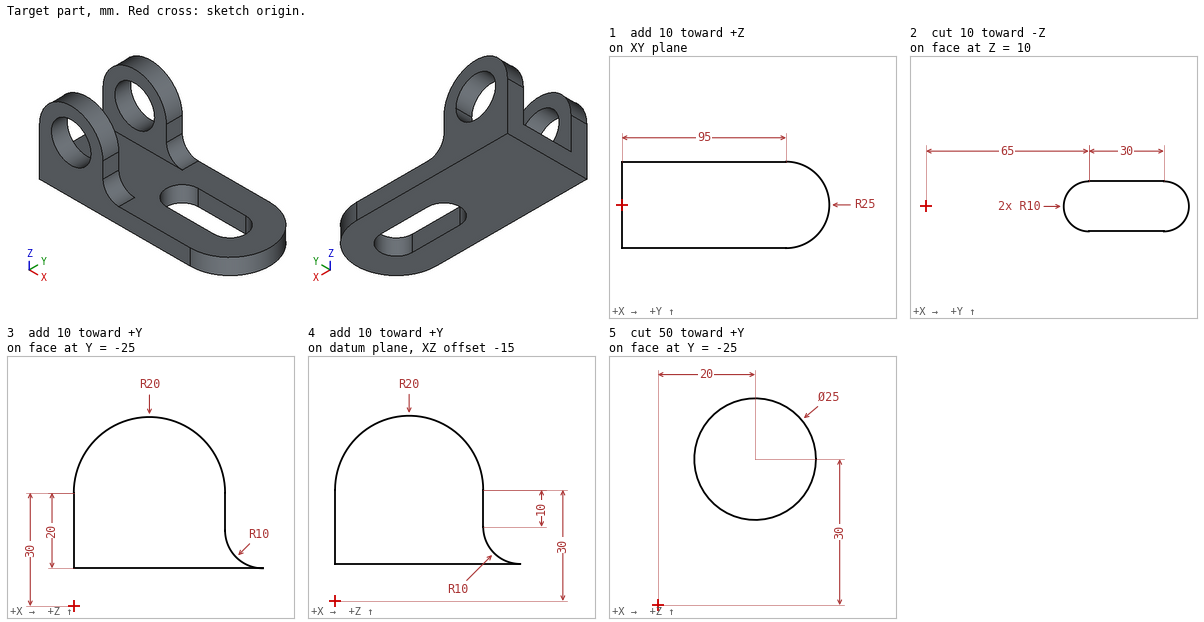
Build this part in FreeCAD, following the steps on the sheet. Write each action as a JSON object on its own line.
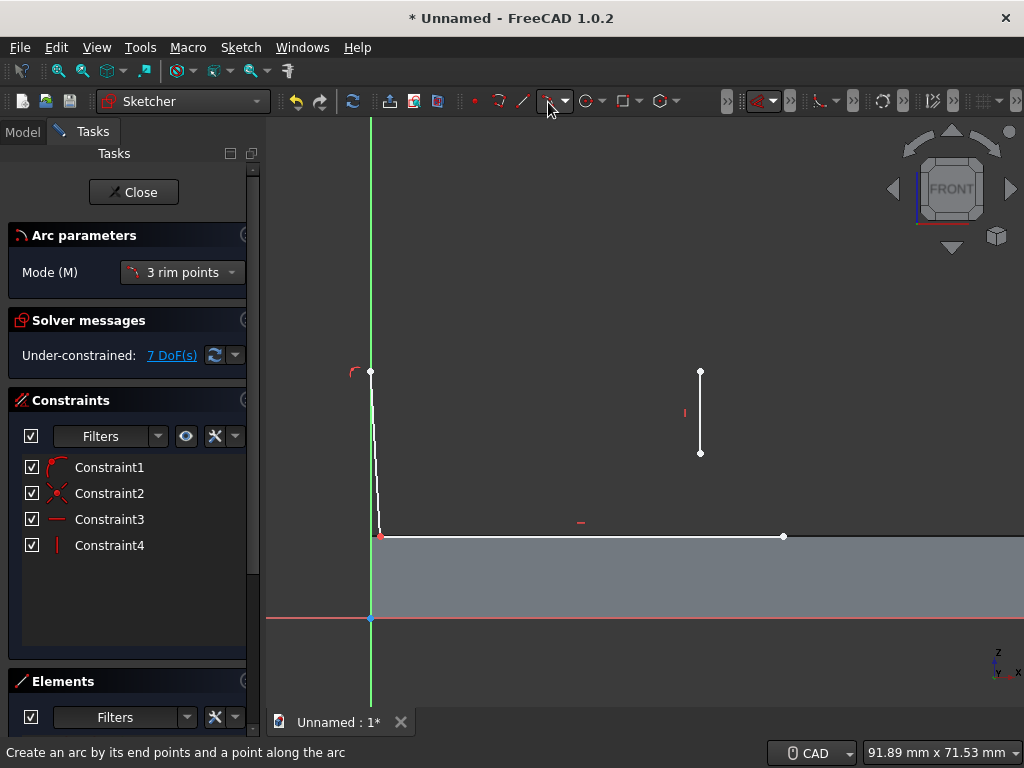
{"action": "left_click", "coordinate": [783, 537]}
{"action": "left_click", "coordinate": [700, 454]}
{"action": "left_click", "coordinate": [725, 512]}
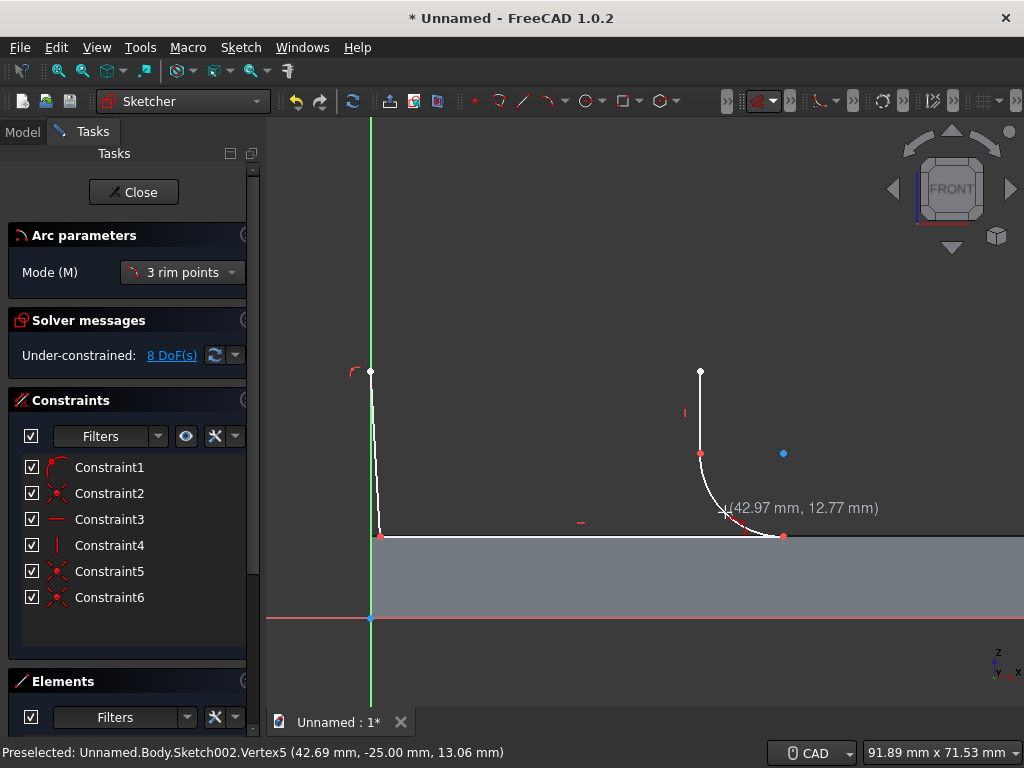
{"action": "left_click", "coordinate": [700, 372]}
{"action": "left_click", "coordinate": [371, 372]}
{"action": "left_click", "coordinate": [536, 206]}
{"action": "key", "text": "Escape"}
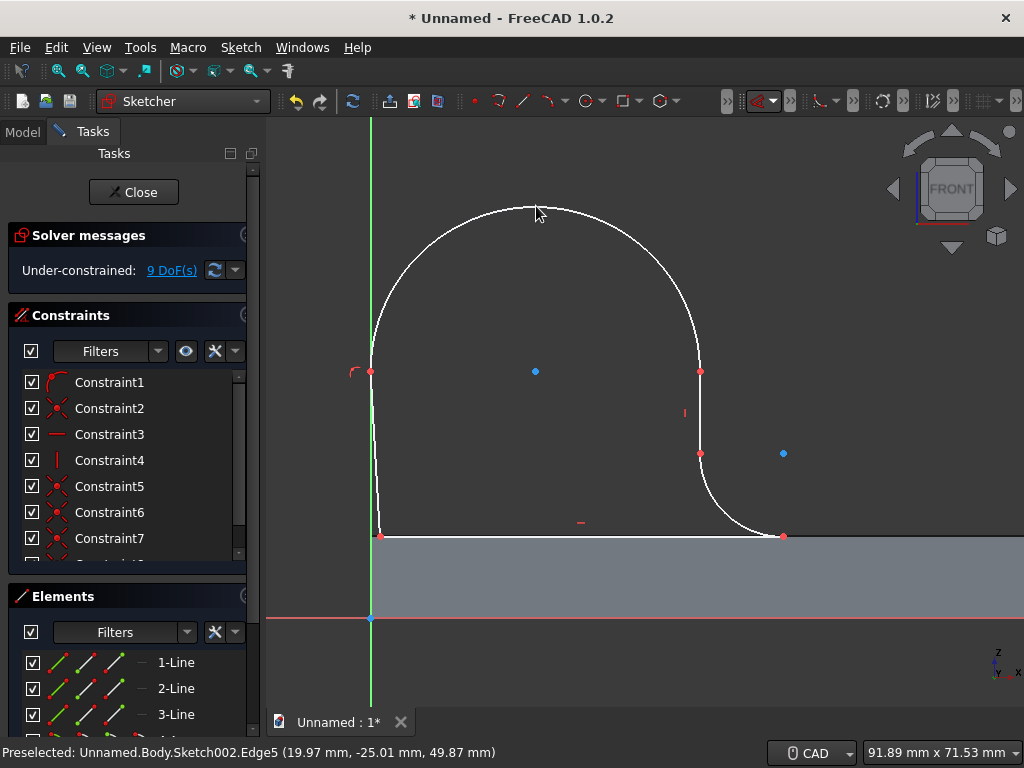
{"action": "left_click", "coordinate": [373, 422]}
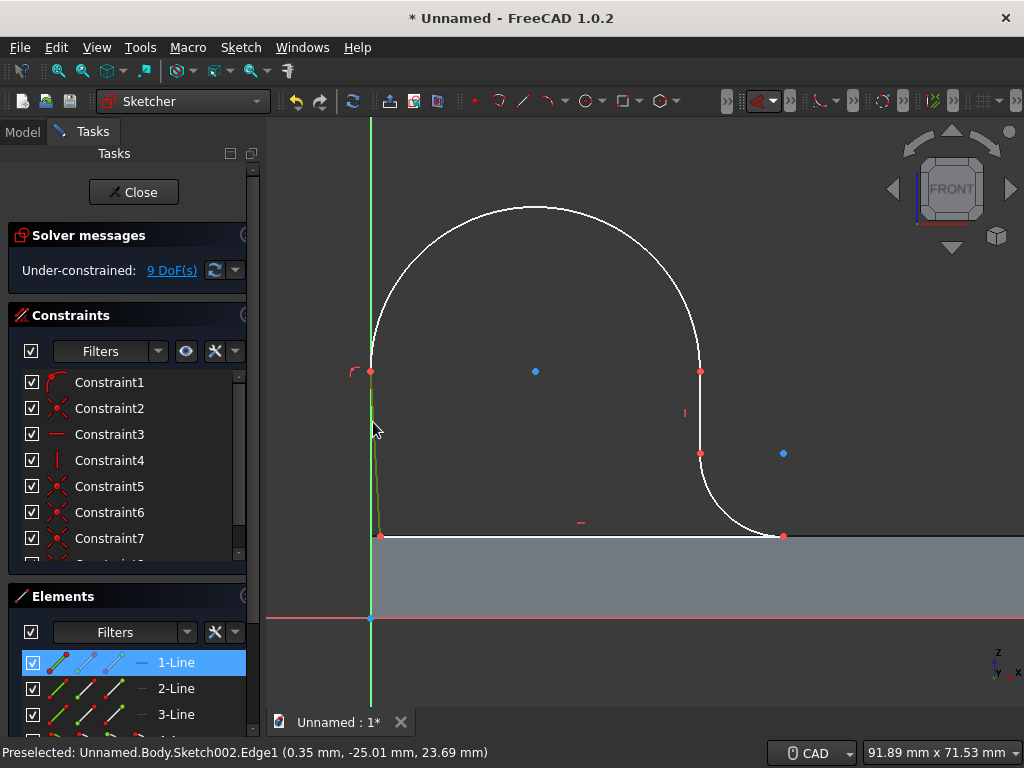
{"action": "left_click", "coordinate": [632, 239]}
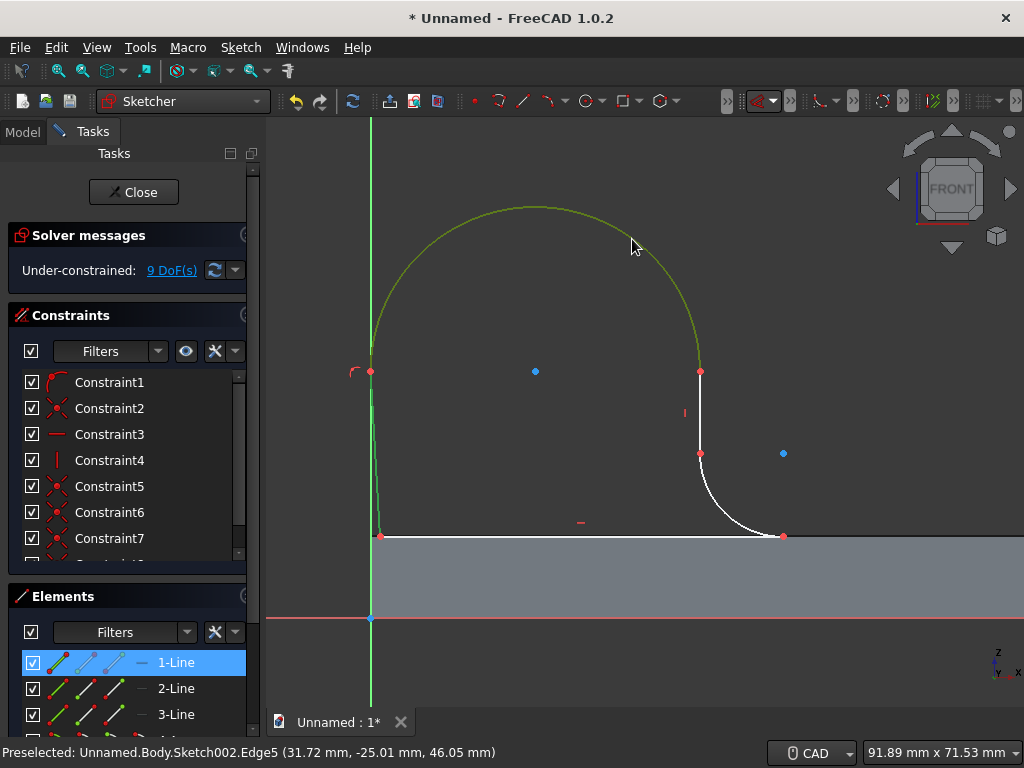
{"action": "key", "text": "t"}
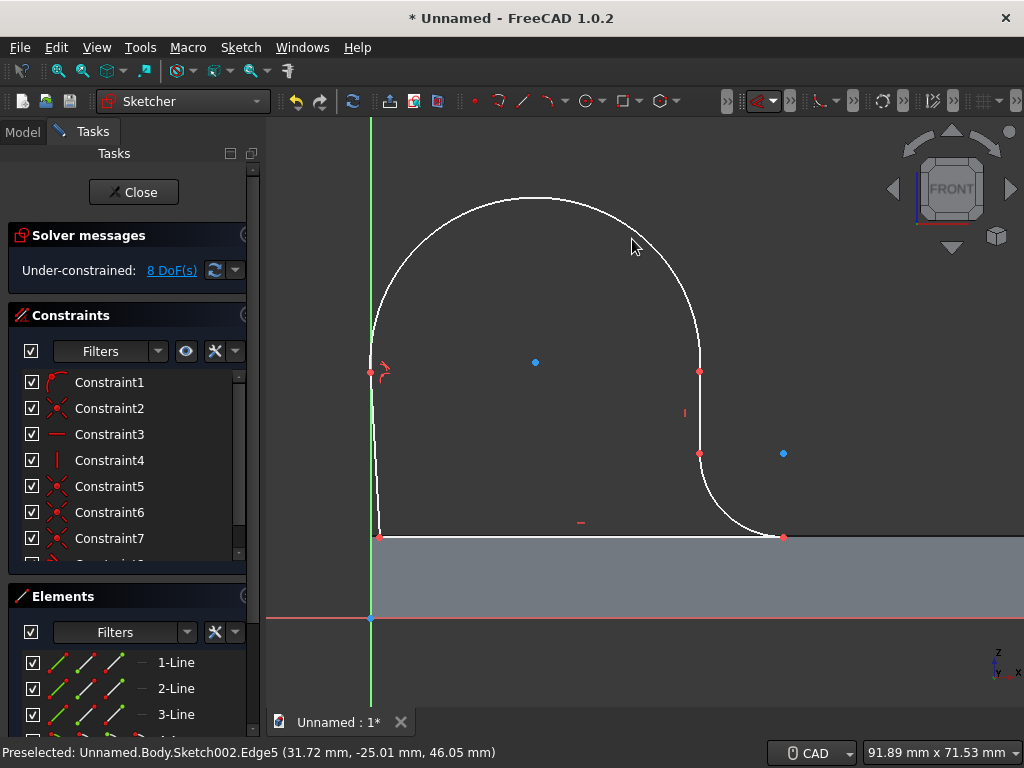
{"action": "left_click", "coordinate": [501, 537]}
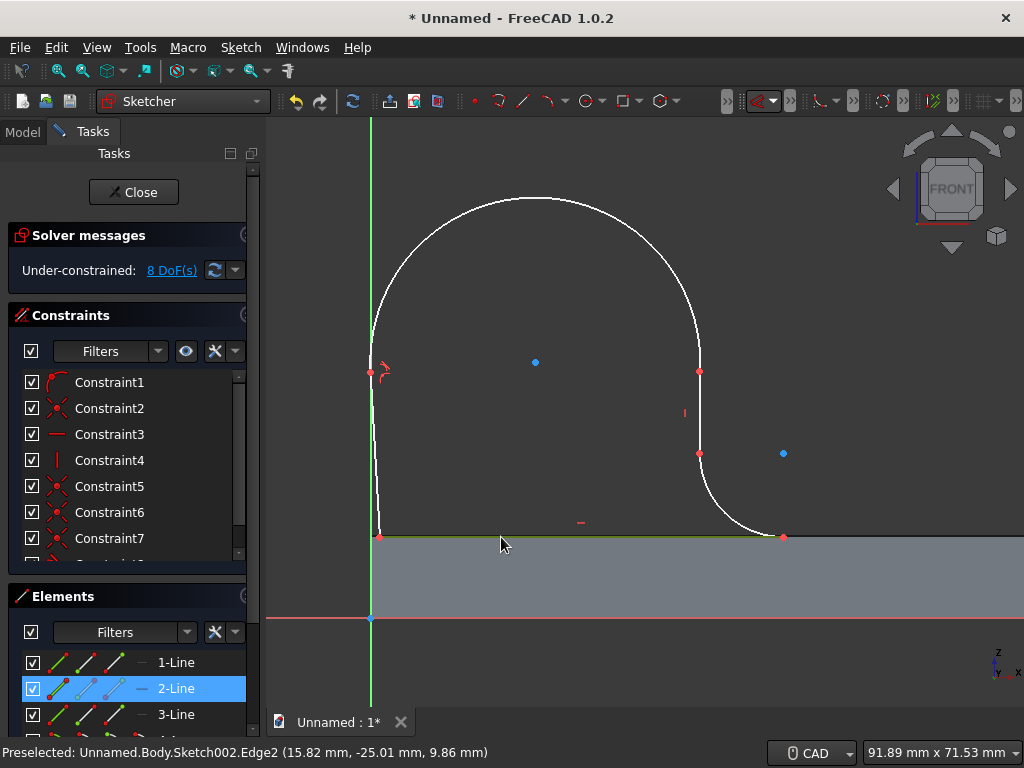
{"action": "left_click", "coordinate": [709, 492]}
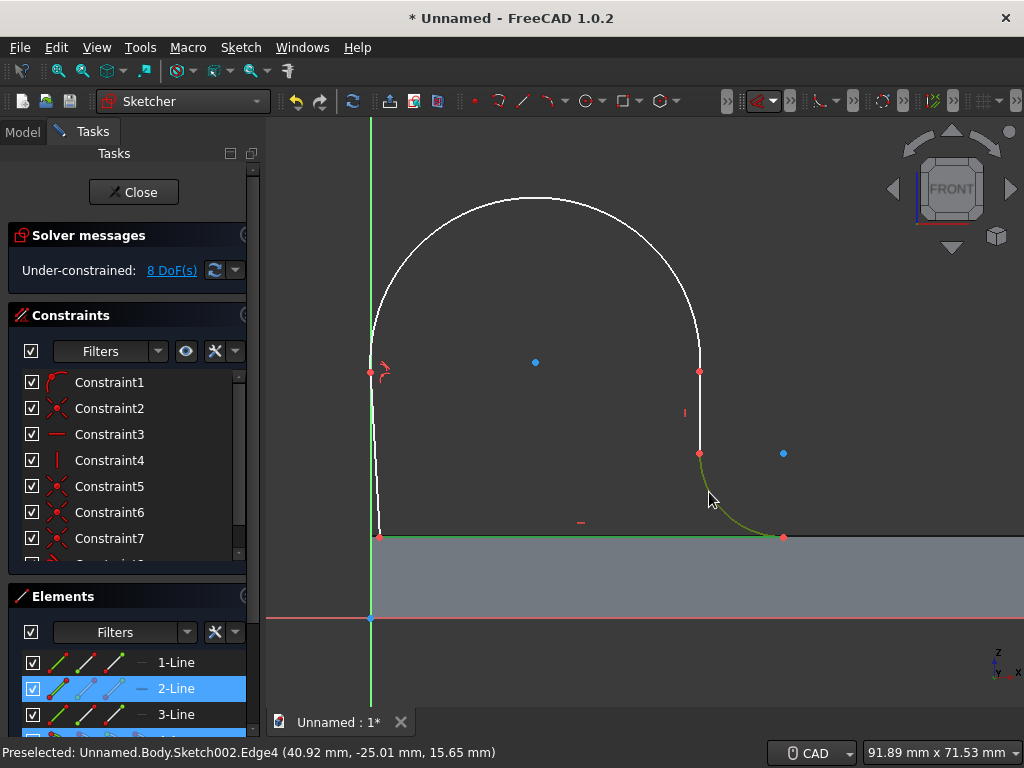
{"action": "key", "text": "t"}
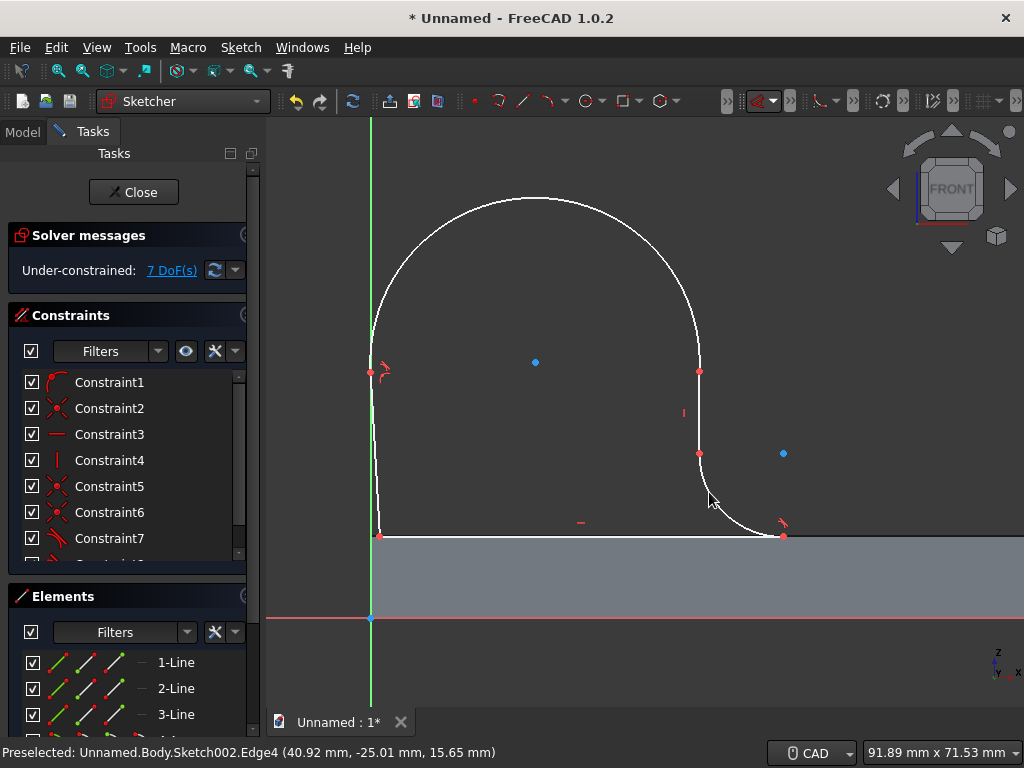
{"action": "left_click", "coordinate": [699, 429]}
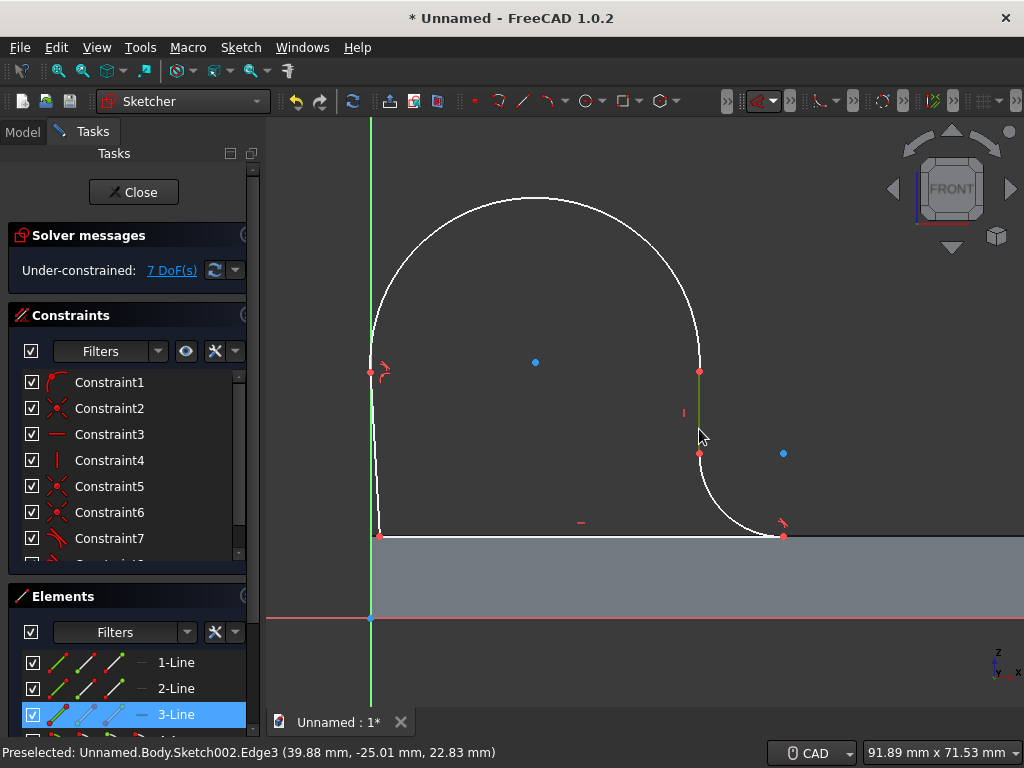
{"action": "left_click", "coordinate": [709, 492]}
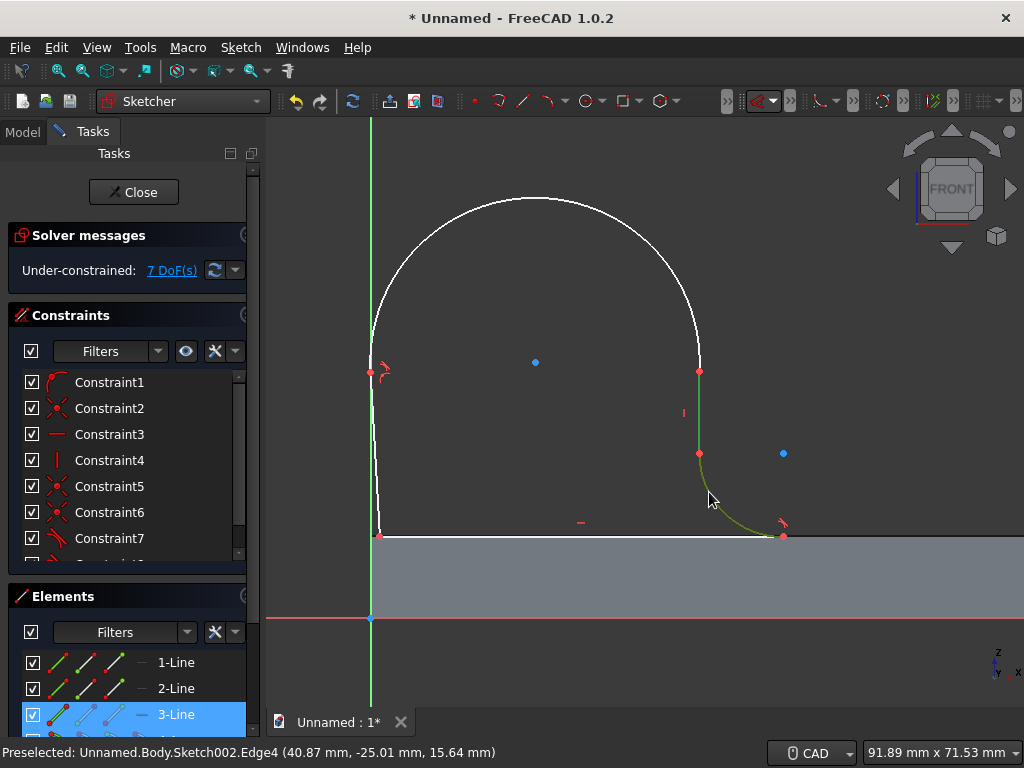
{"action": "key", "text": "t"}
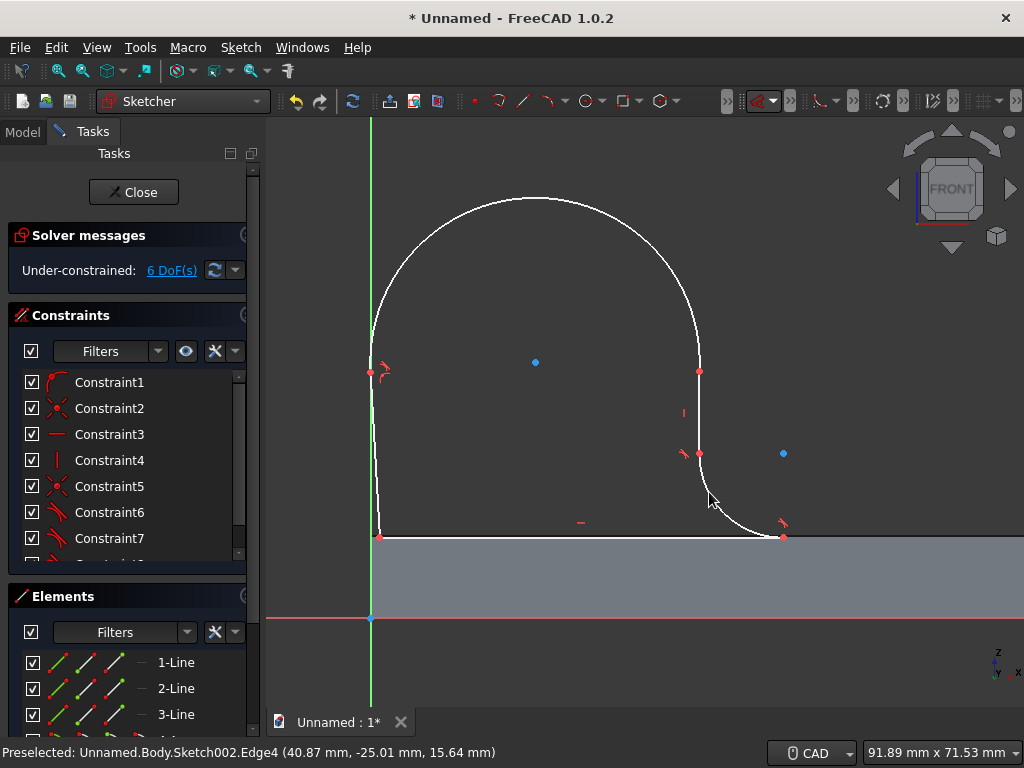
{"action": "left_click", "coordinate": [699, 429]}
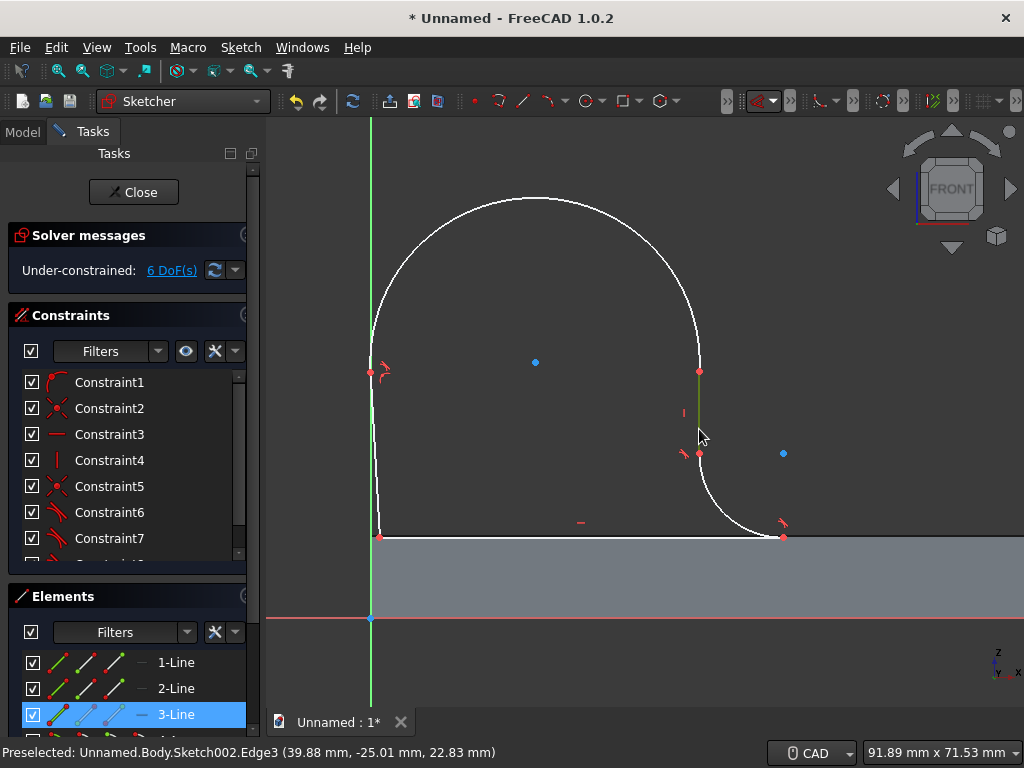
{"action": "left_click", "coordinate": [635, 232]}